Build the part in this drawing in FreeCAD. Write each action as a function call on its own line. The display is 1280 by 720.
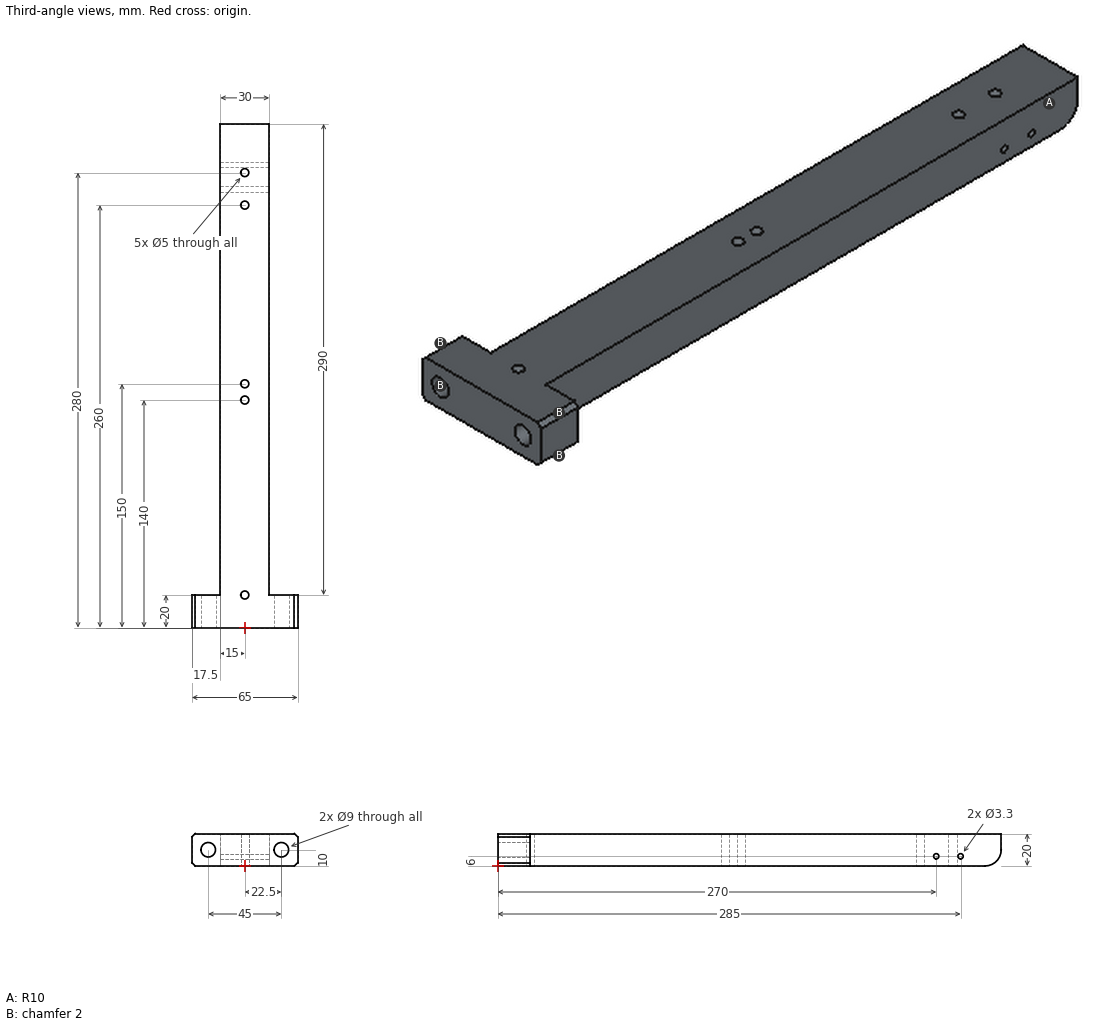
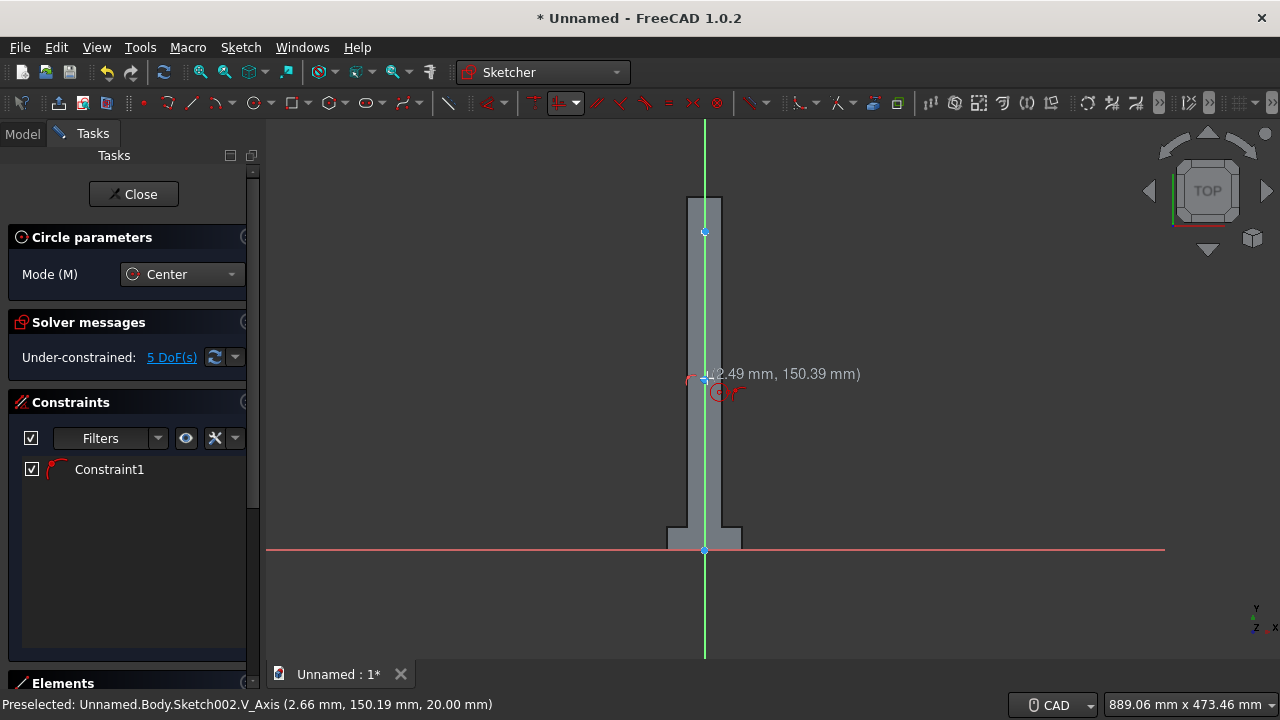
scroll(705, 527, up, 11)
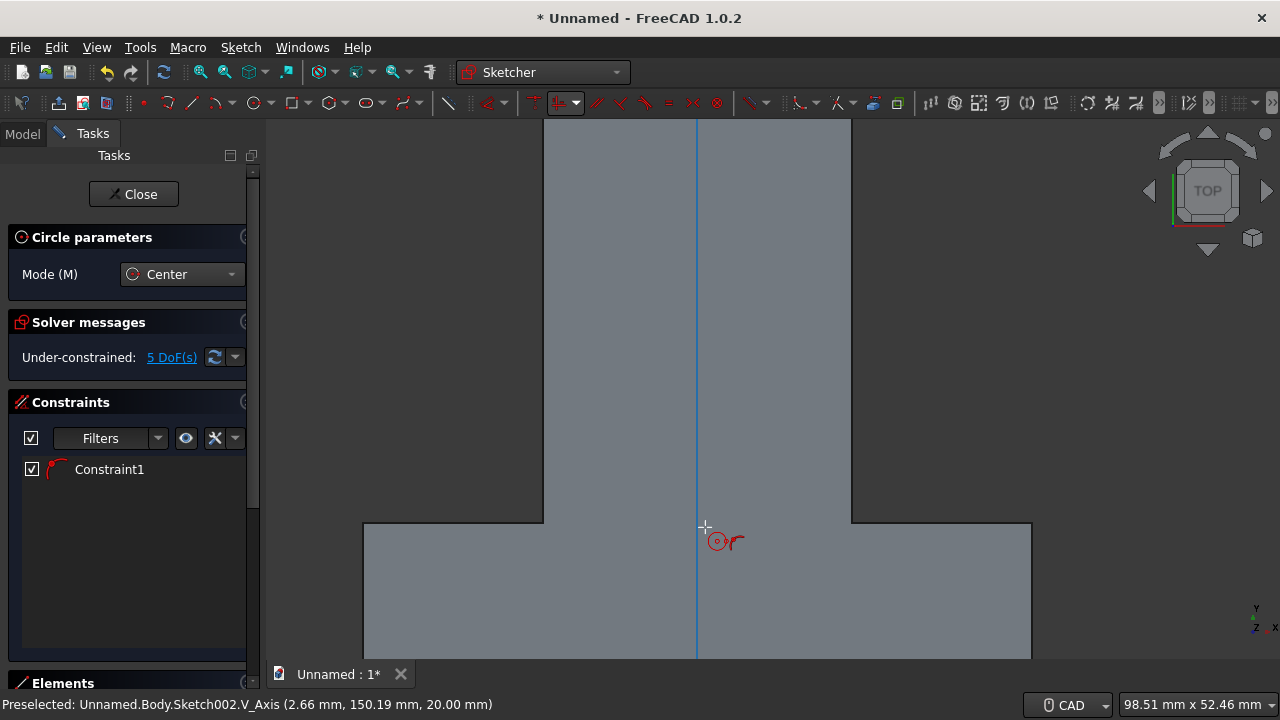
scroll(705, 528, down, 11)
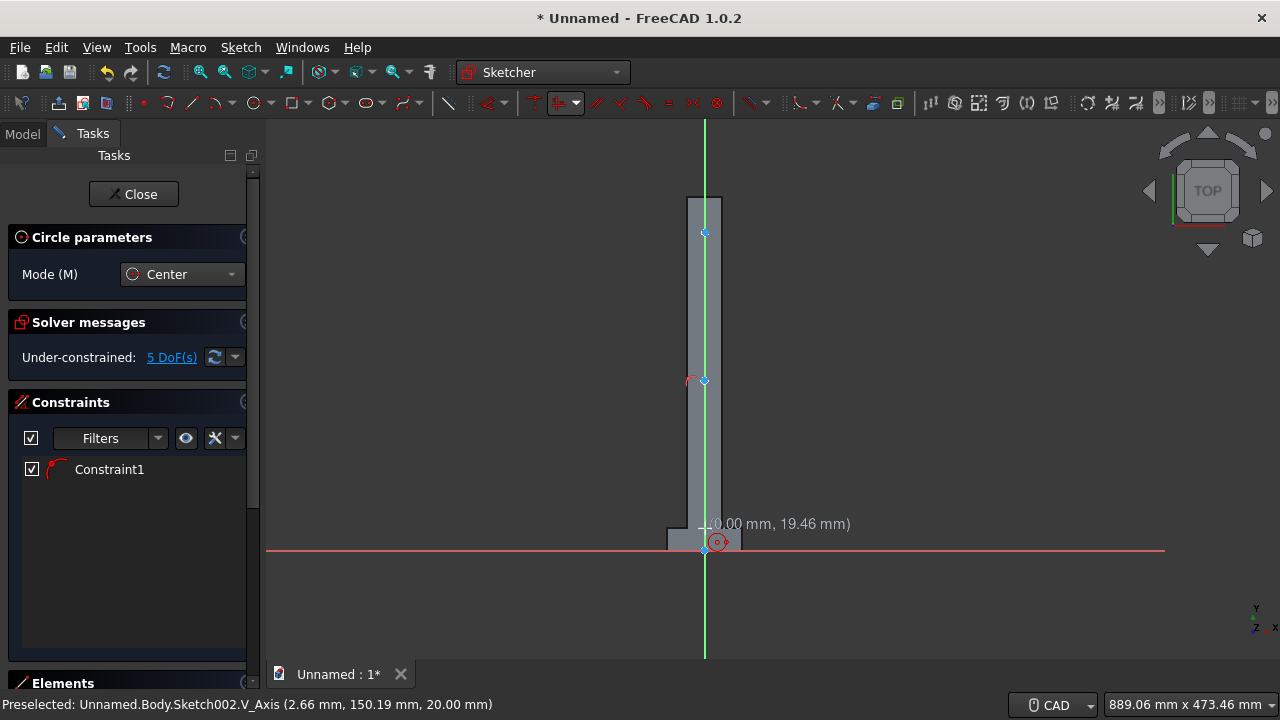
click(705, 528)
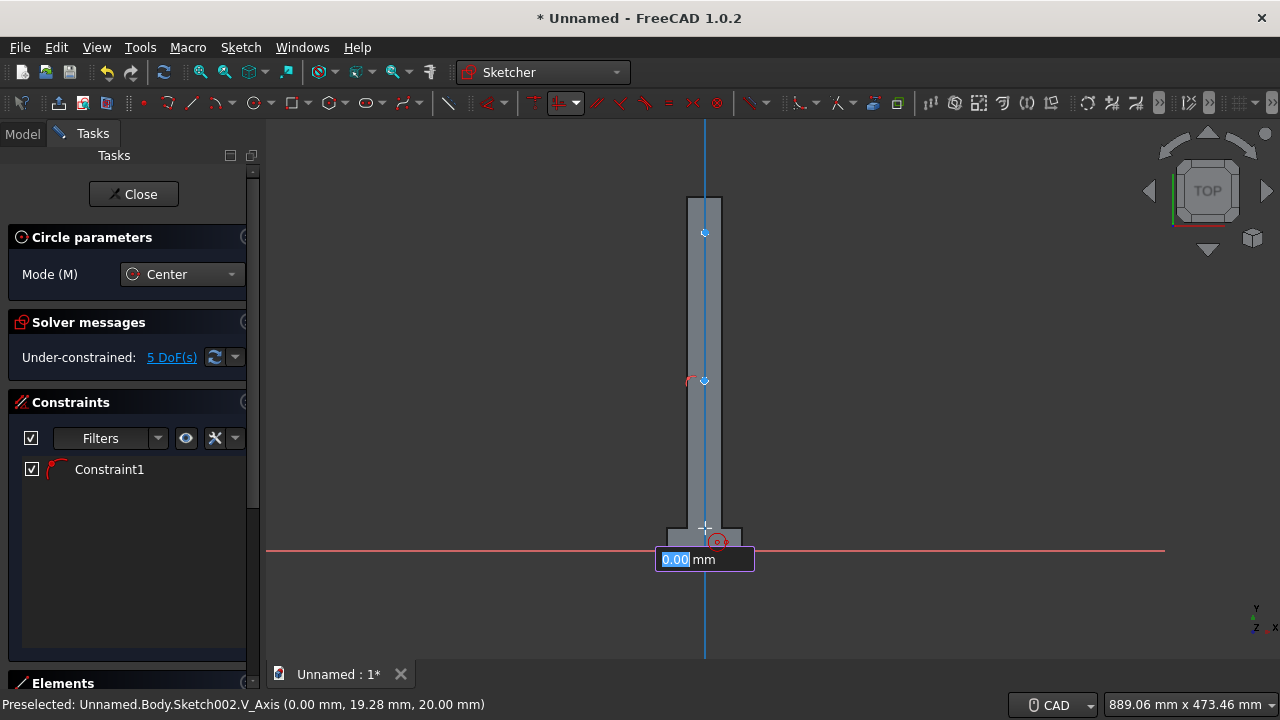
scroll(707, 527, up, 9)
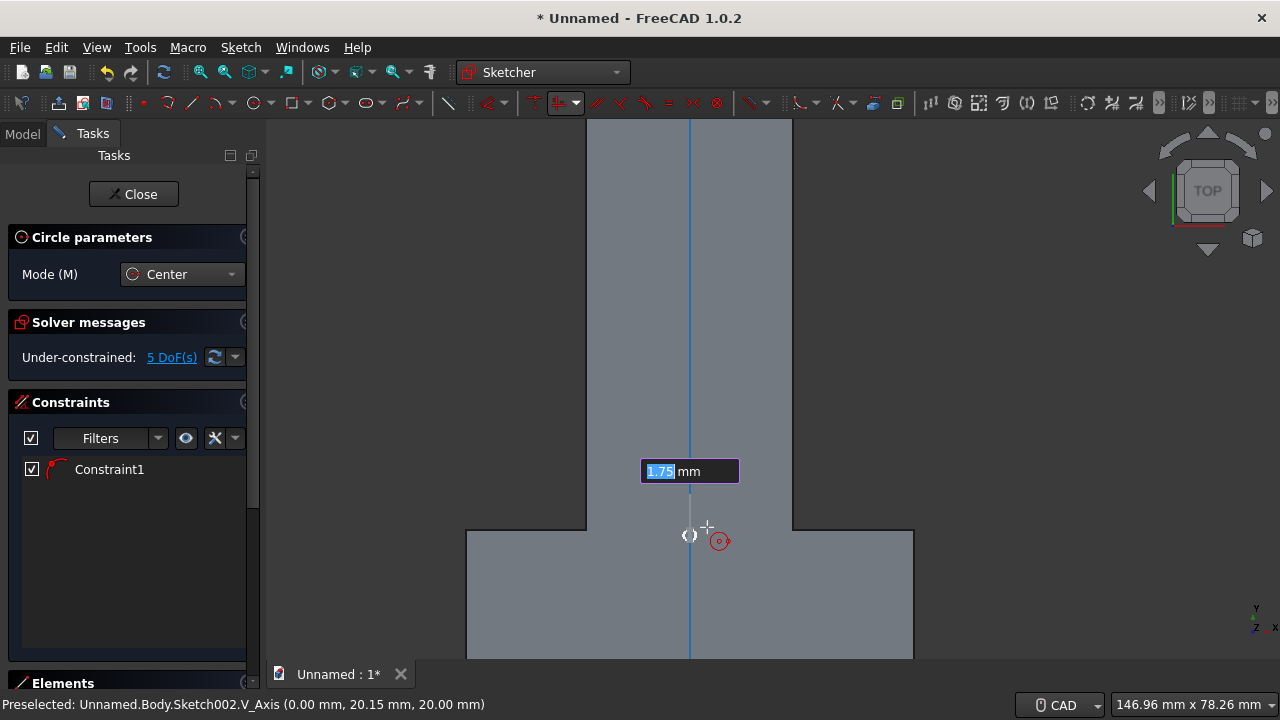
click(706, 524)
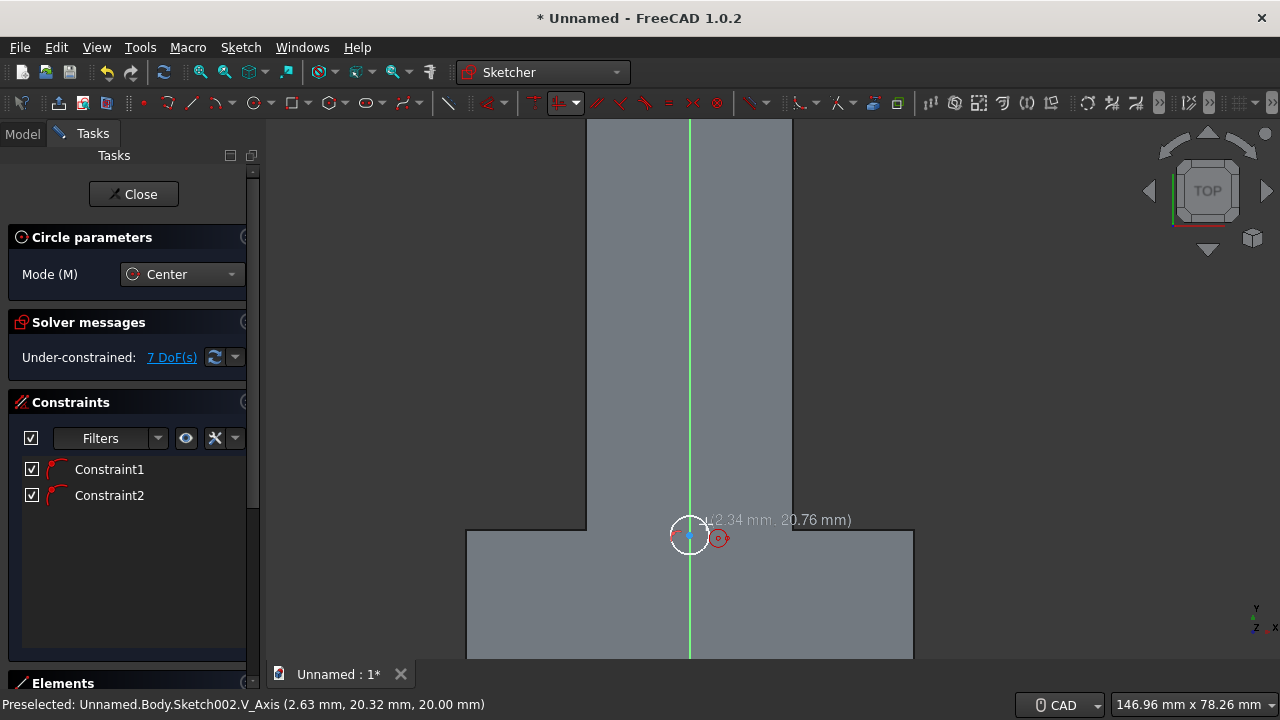
scroll(707, 527, down, 9)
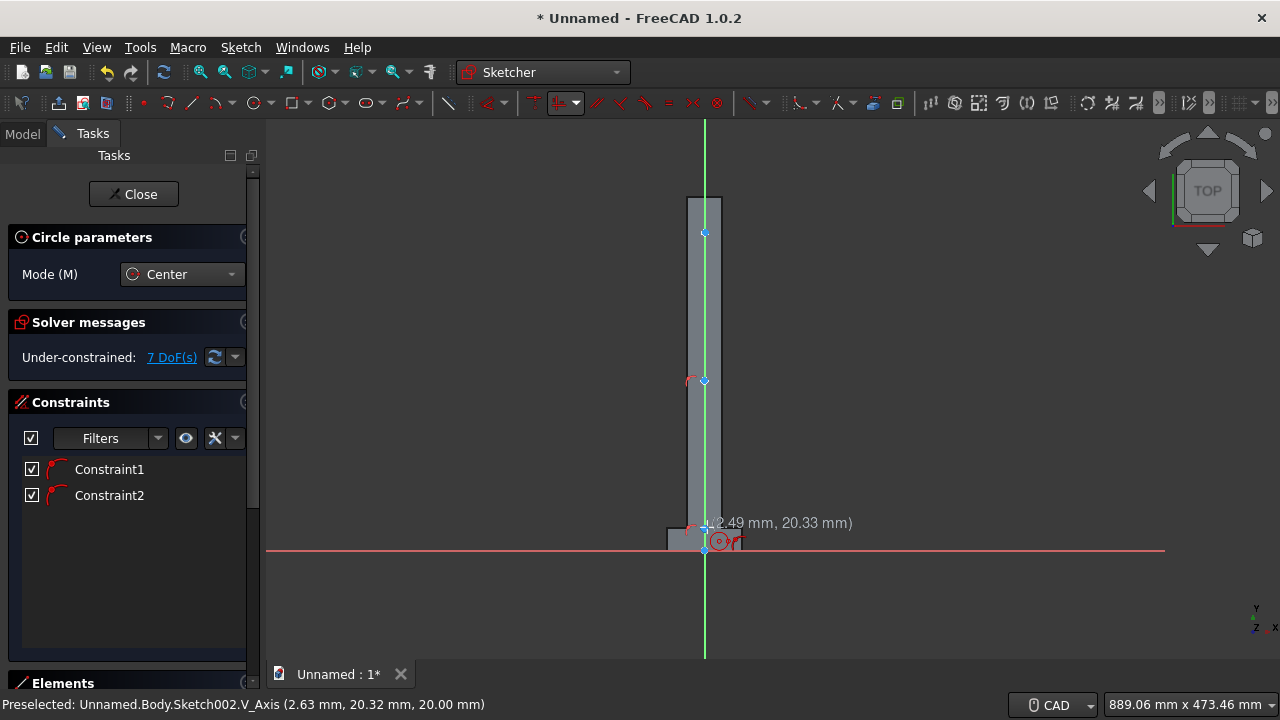
scroll(705, 254, up, 11)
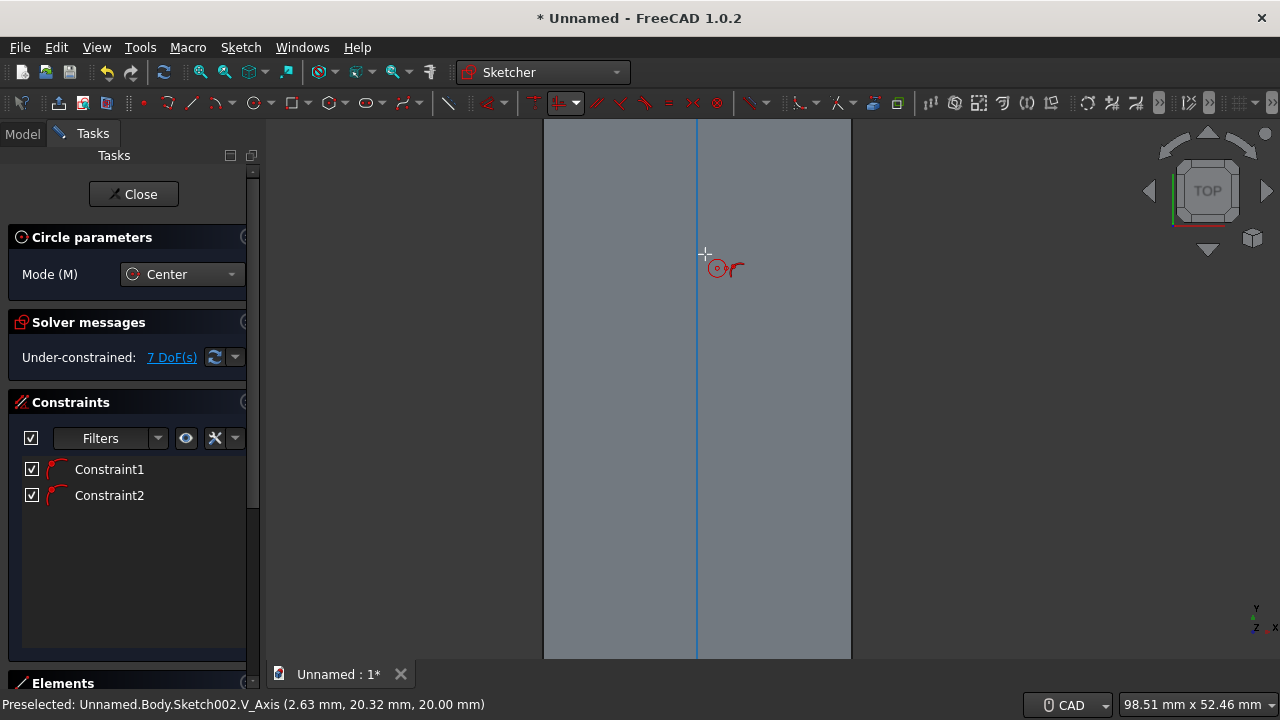
scroll(705, 253, down, 11)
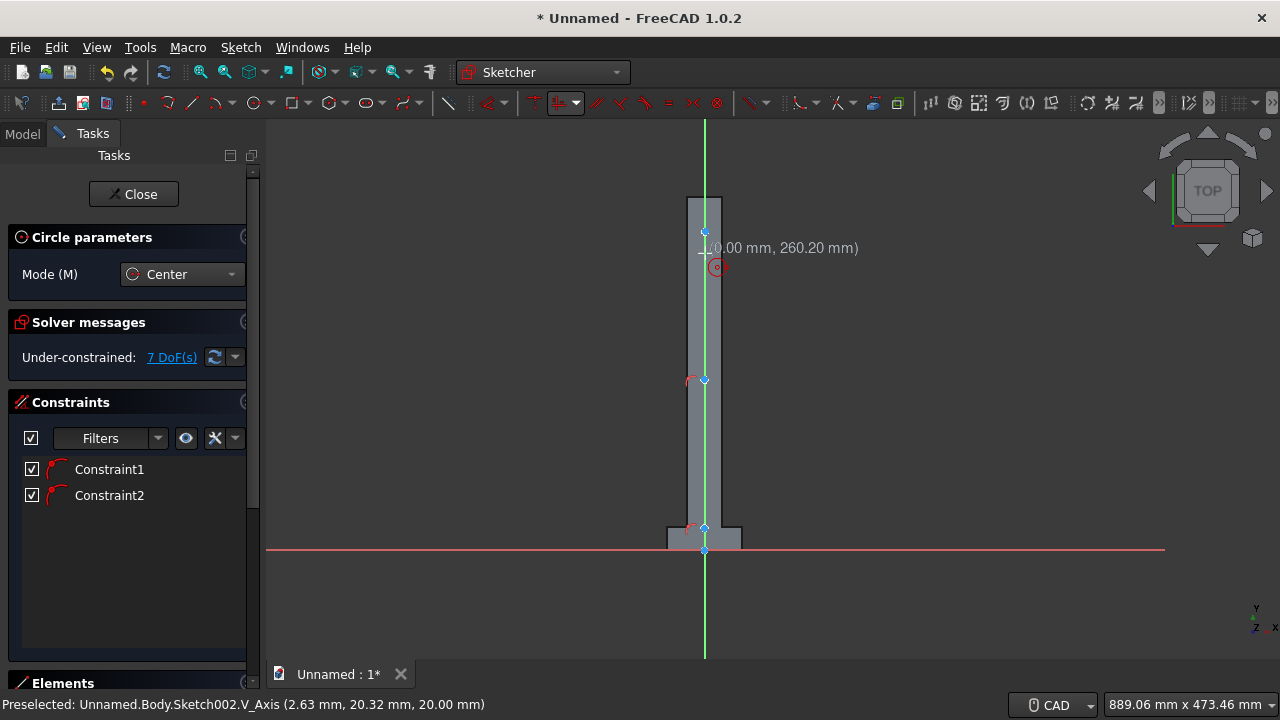
click(705, 254)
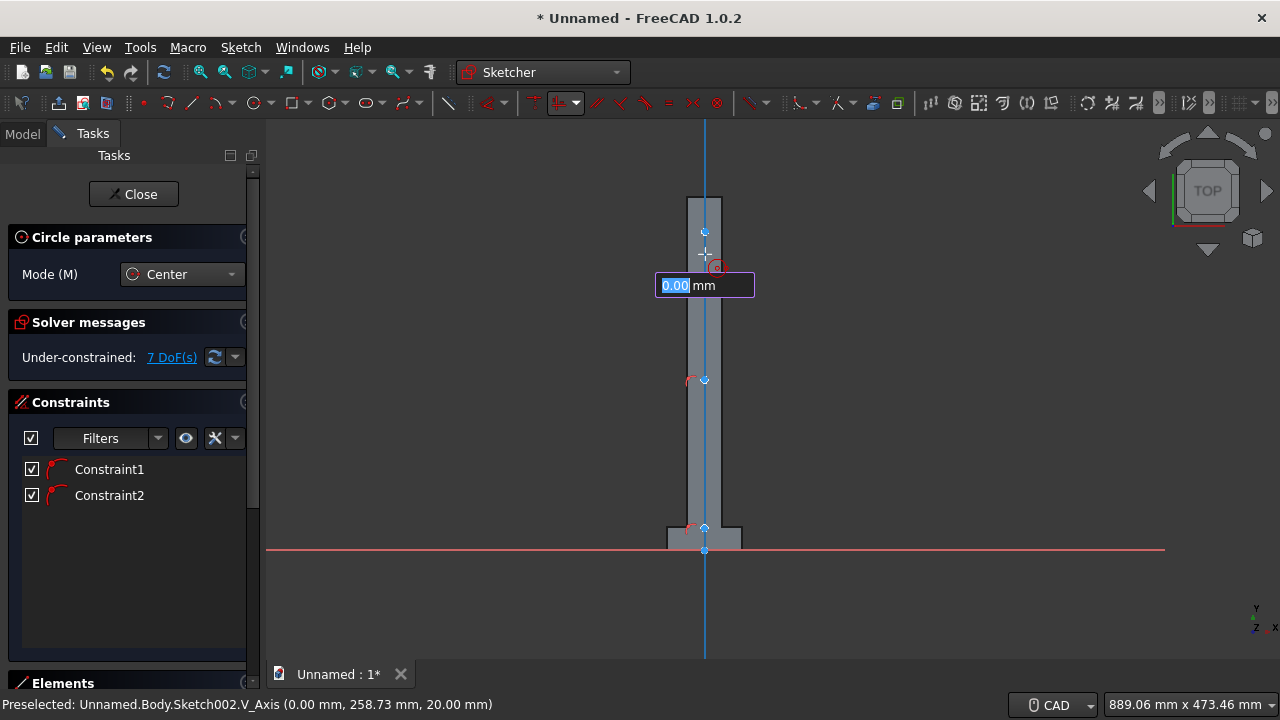
scroll(707, 253, up, 9)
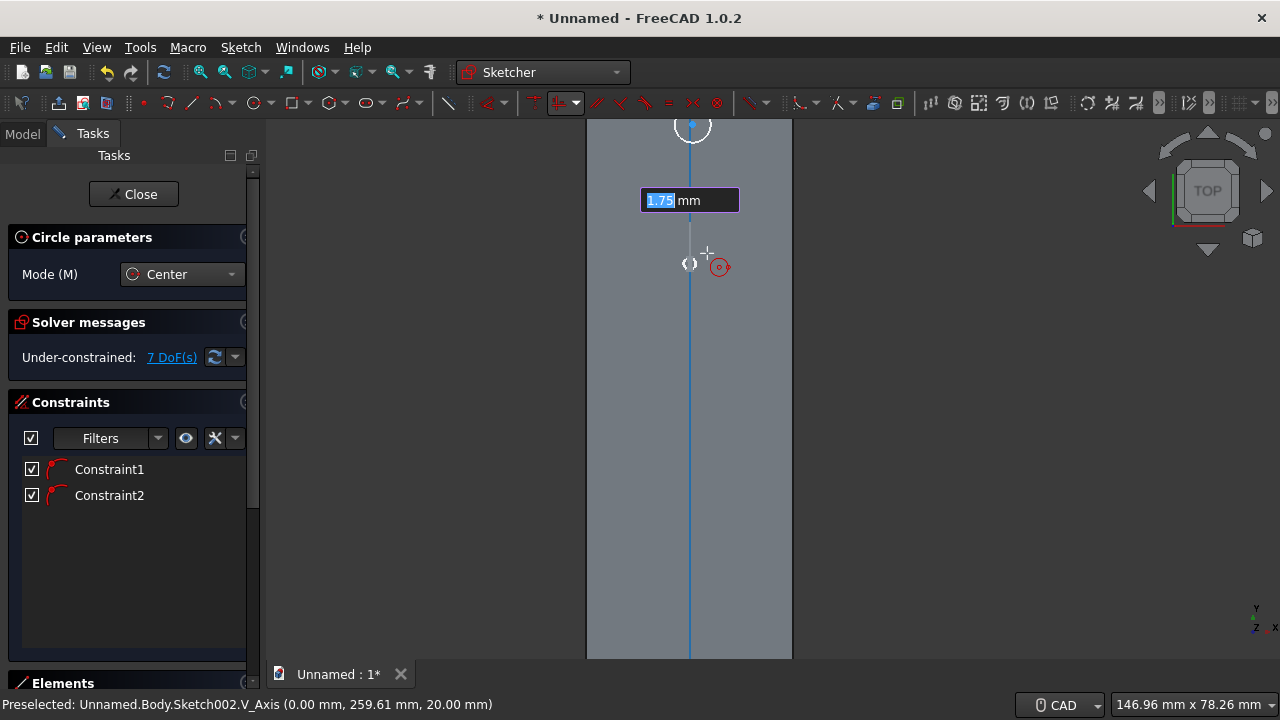
click(706, 249)